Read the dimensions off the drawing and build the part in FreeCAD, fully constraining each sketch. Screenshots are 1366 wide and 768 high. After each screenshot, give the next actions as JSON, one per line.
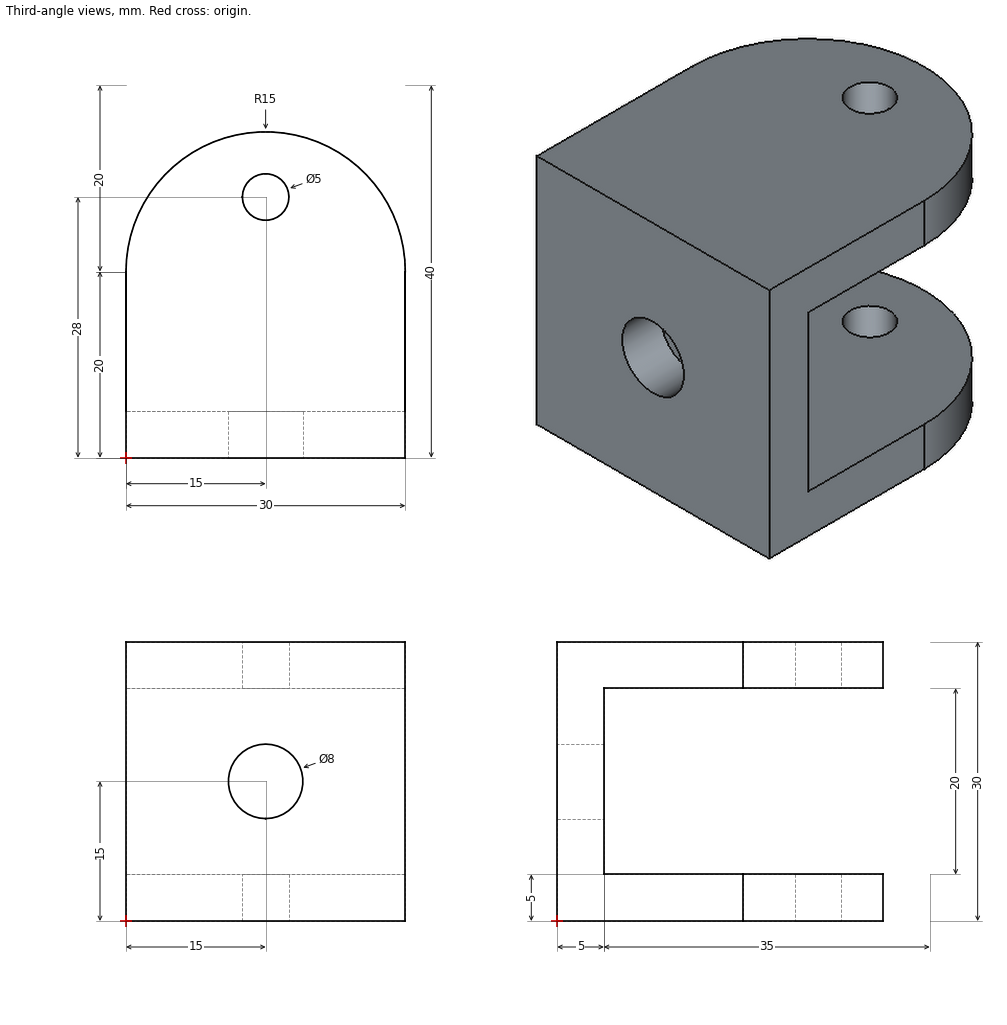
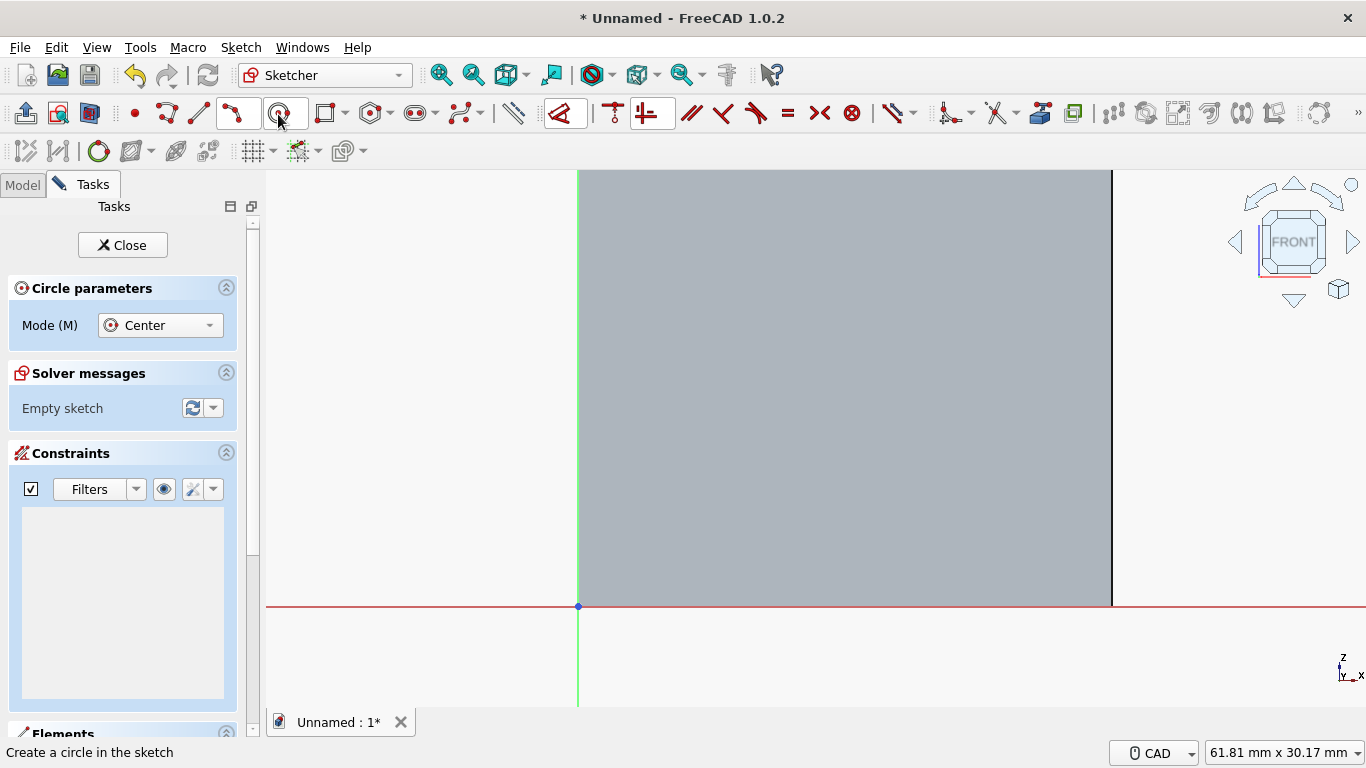
{"action": "left_click", "coordinate": [845, 340]}
{"action": "mouse_move", "coordinate": [896, 289]}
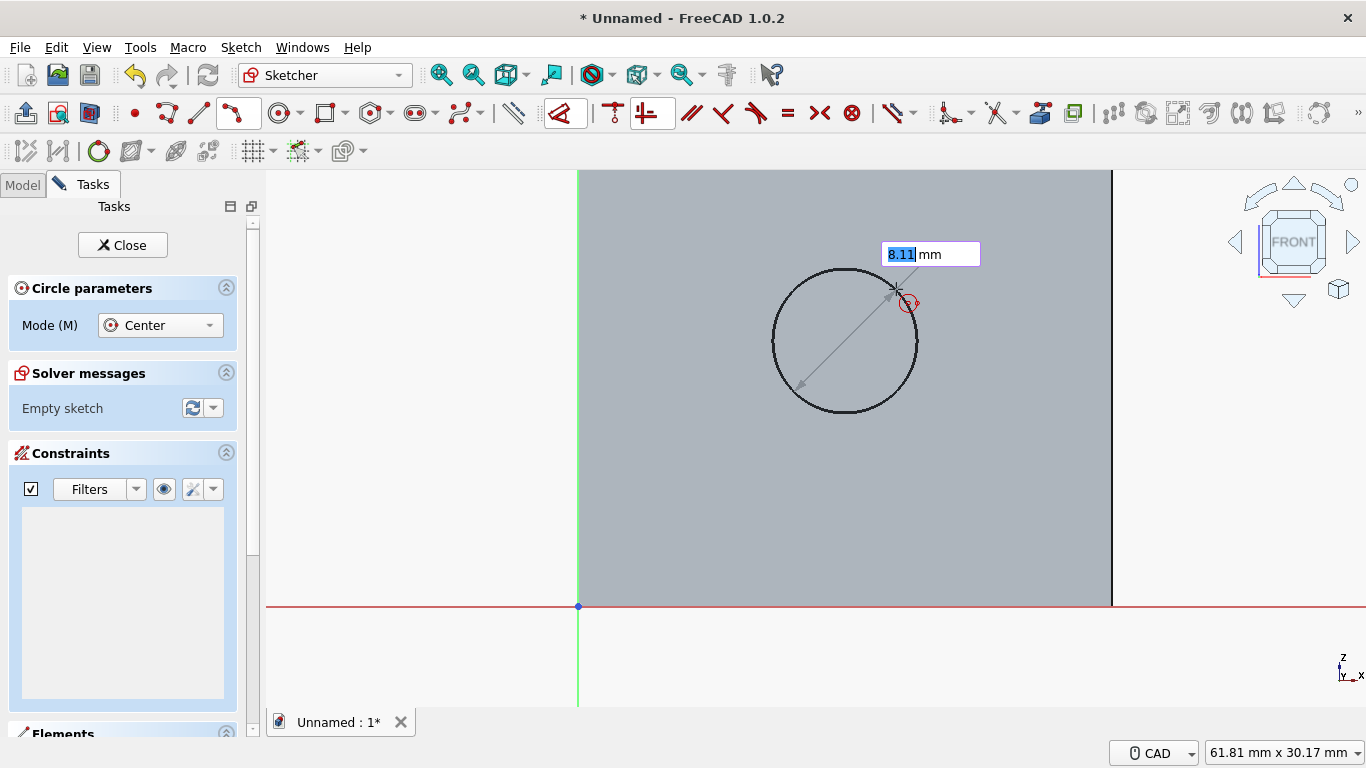
{"action": "type", "text": "8"}
{"action": "key", "text": "Return"}
{"action": "key", "text": "Escape"}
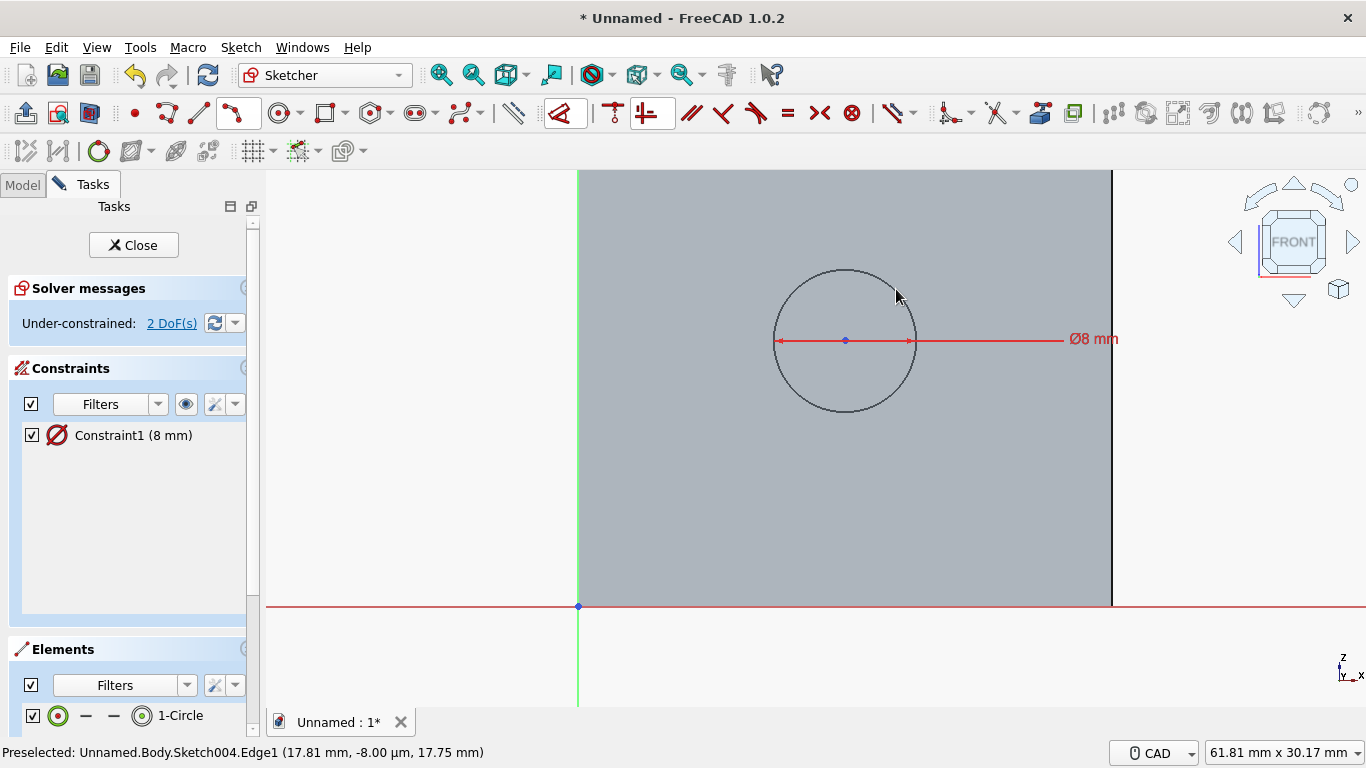
{"action": "left_click", "coordinate": [845, 341]}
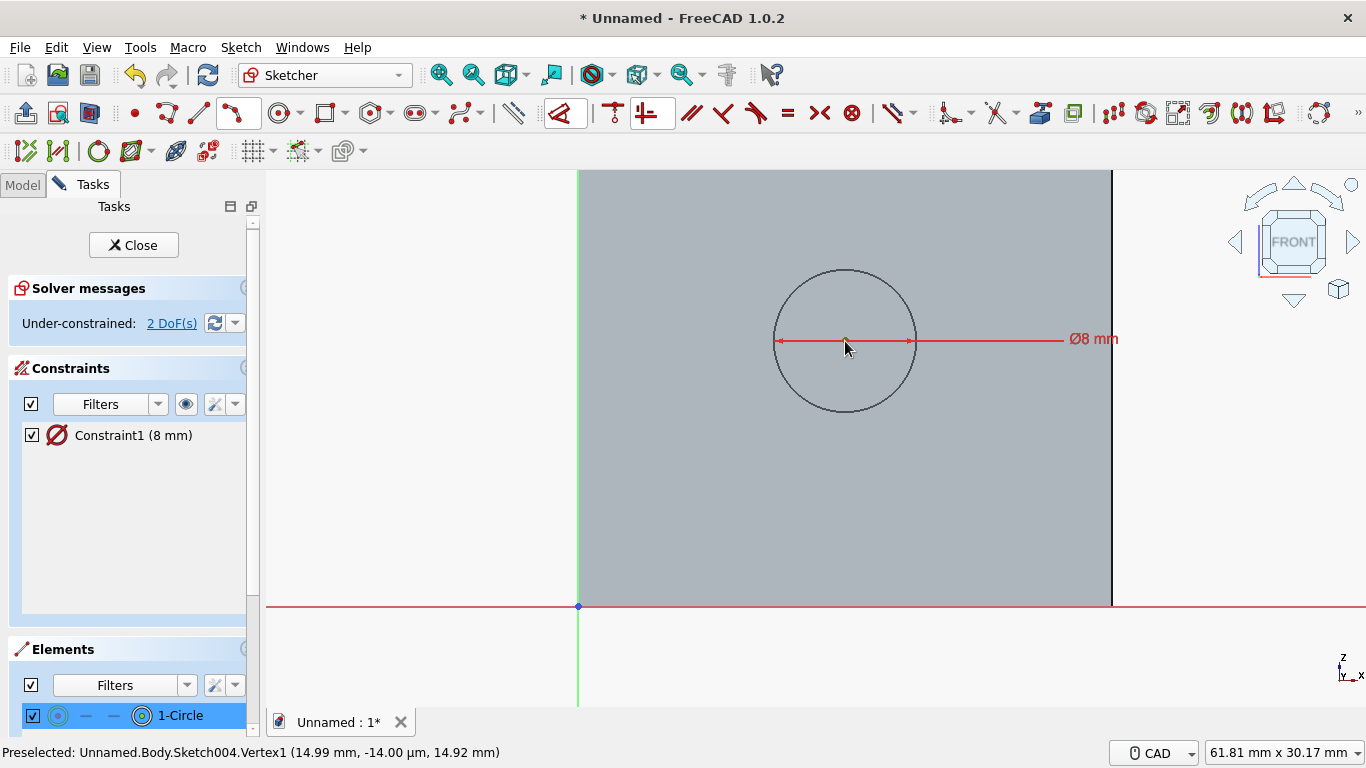
{"action": "key", "text": "l"}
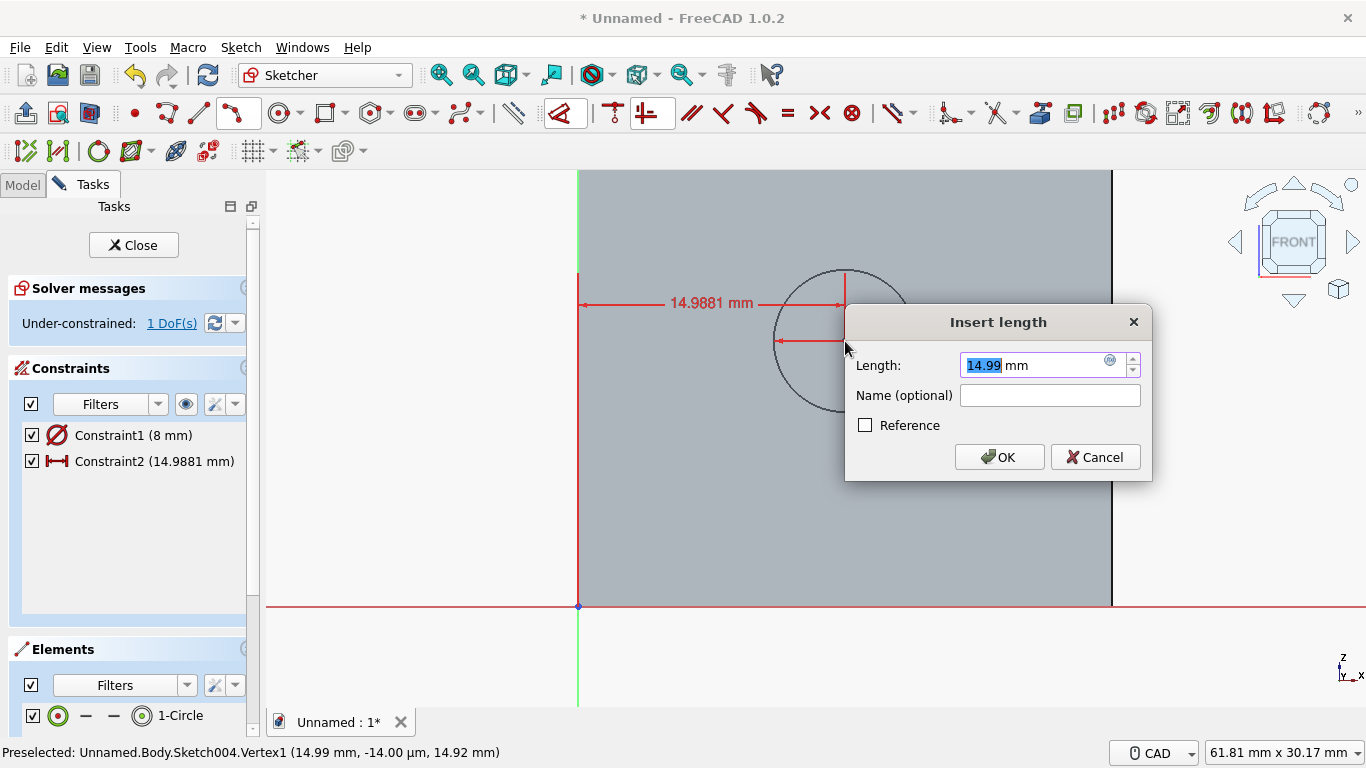
{"action": "type", "text": "15"}
{"action": "key", "text": "Return"}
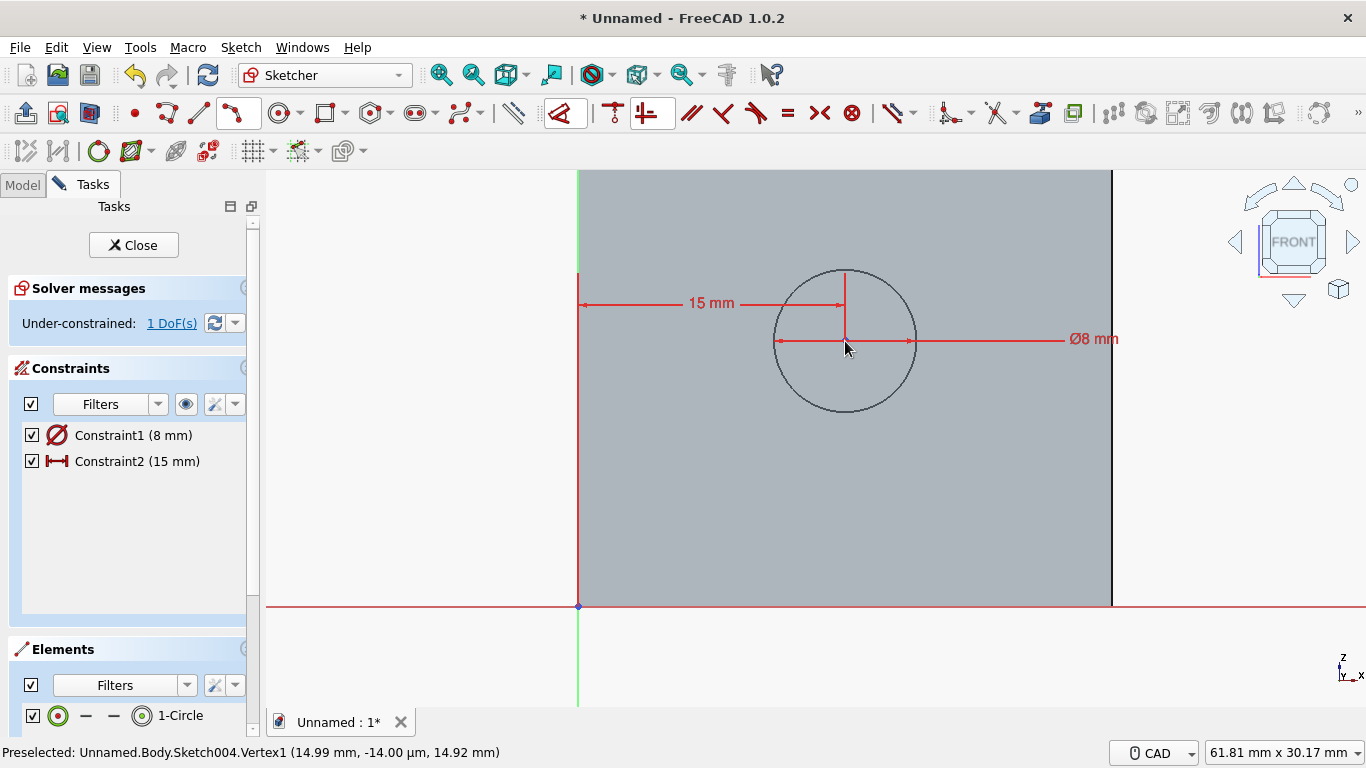
{"action": "left_click", "coordinate": [845, 341]}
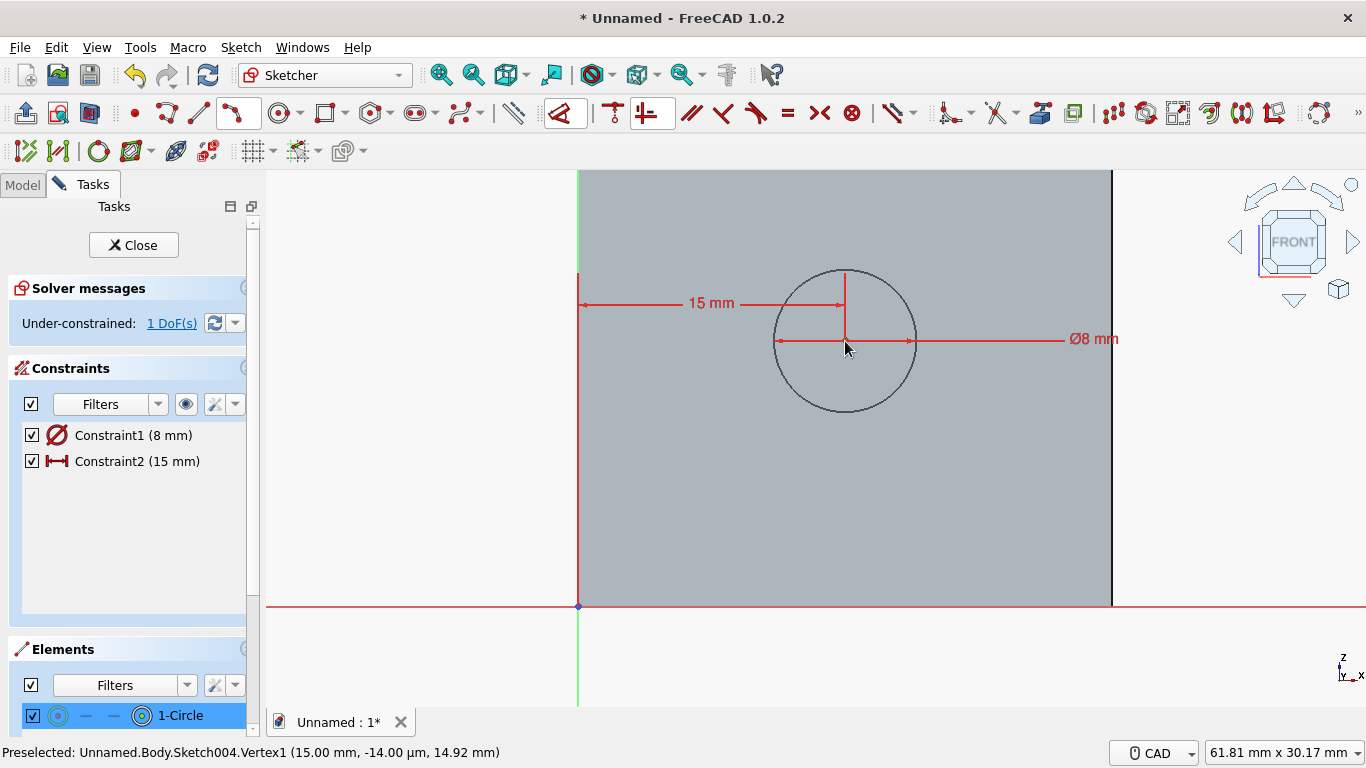
{"action": "key", "text": "i"}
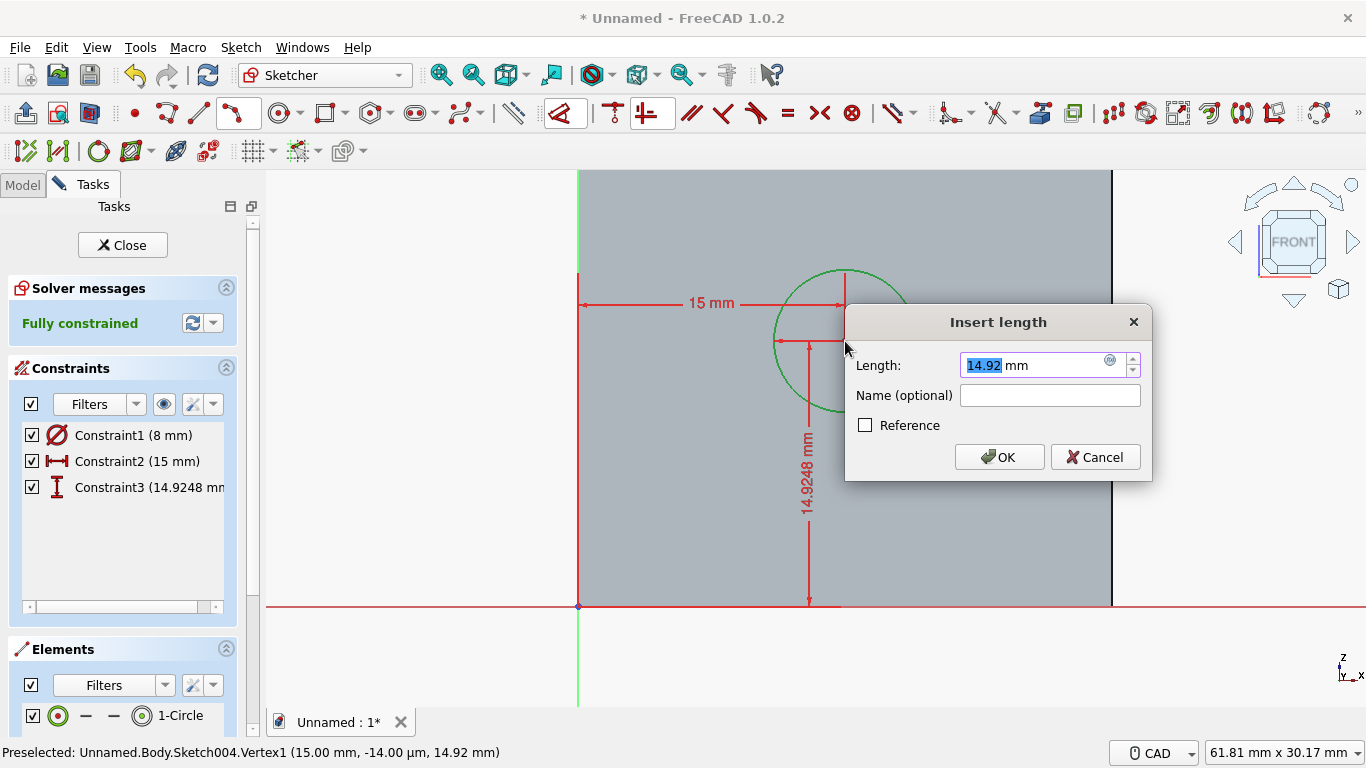
{"action": "type", "text": "15"}
{"action": "key", "text": "Return"}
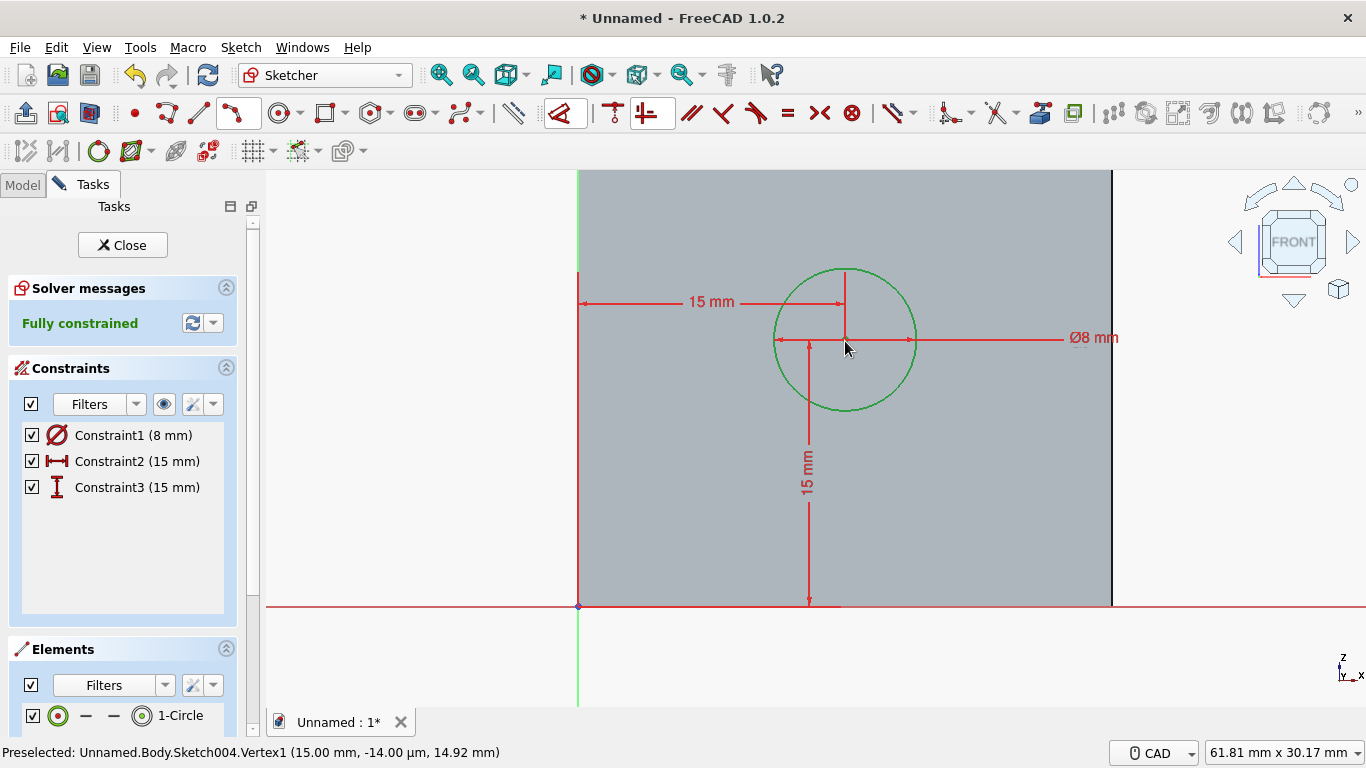
{"action": "left_click", "coordinate": [123, 245]}